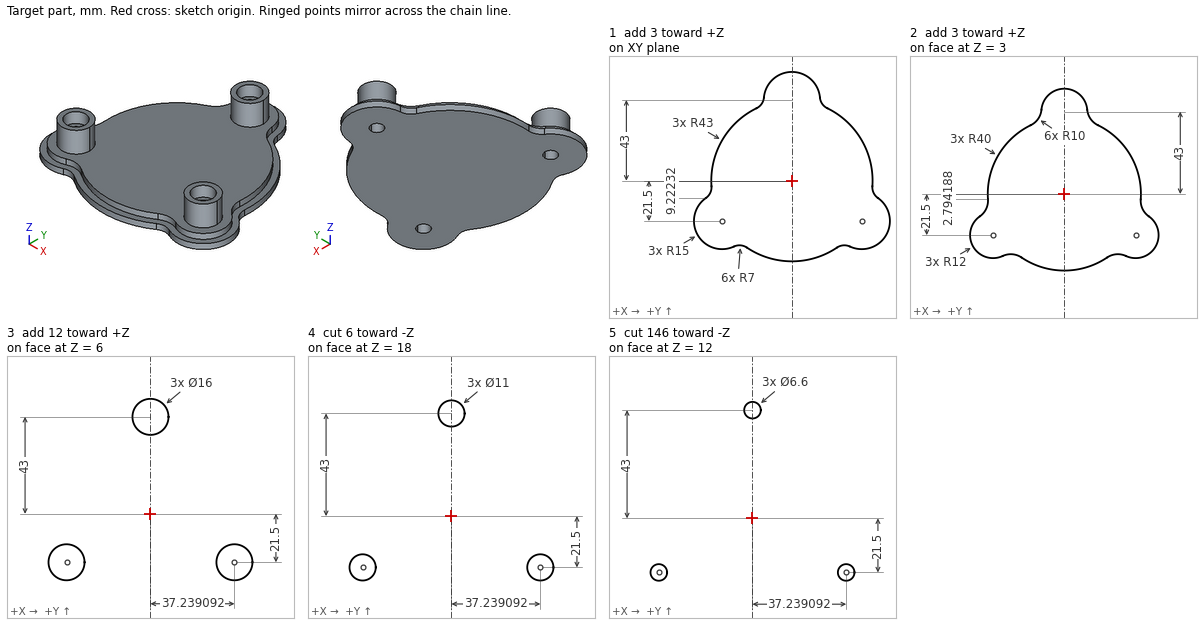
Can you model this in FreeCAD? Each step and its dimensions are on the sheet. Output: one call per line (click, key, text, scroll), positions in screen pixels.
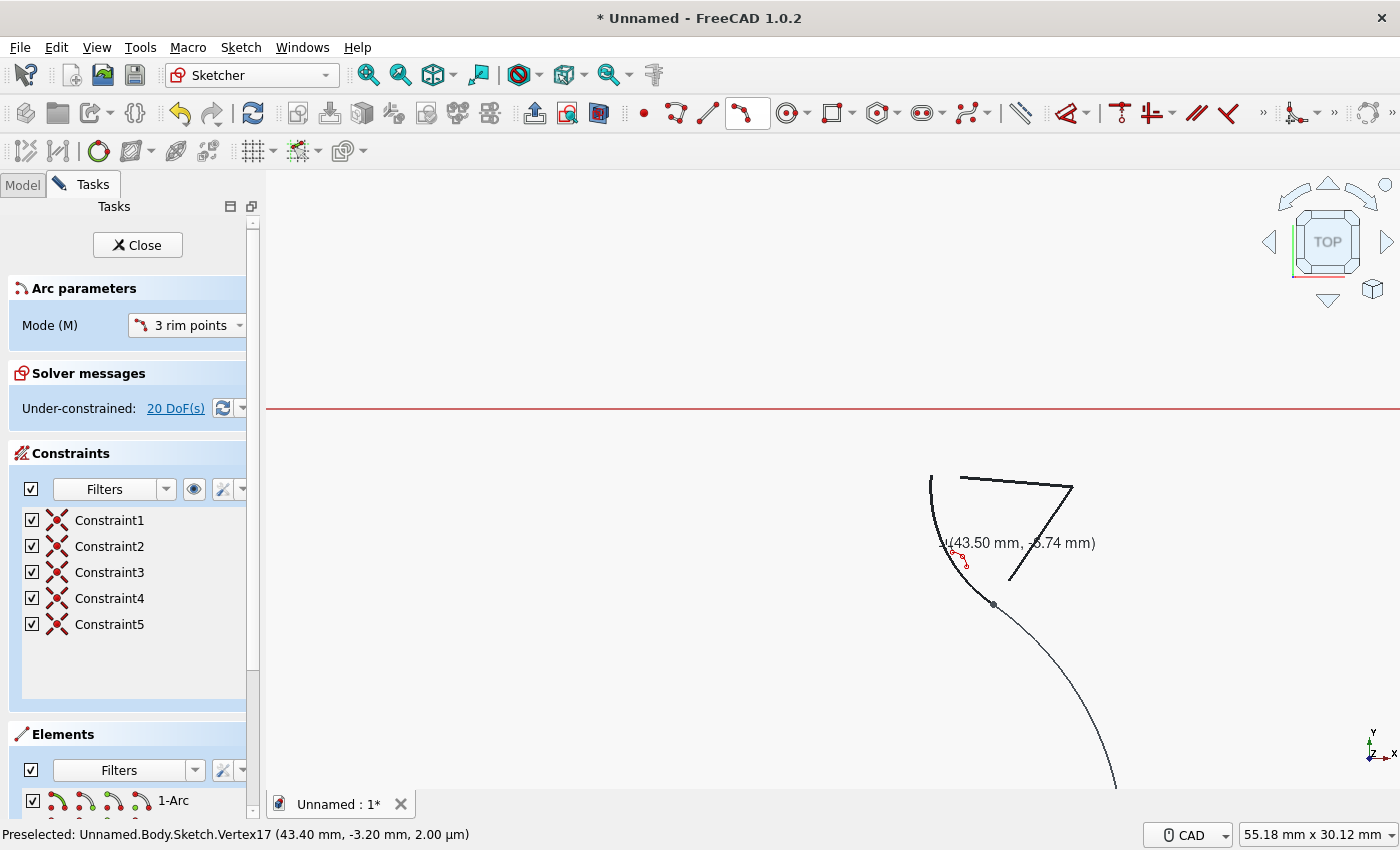
click(946, 543)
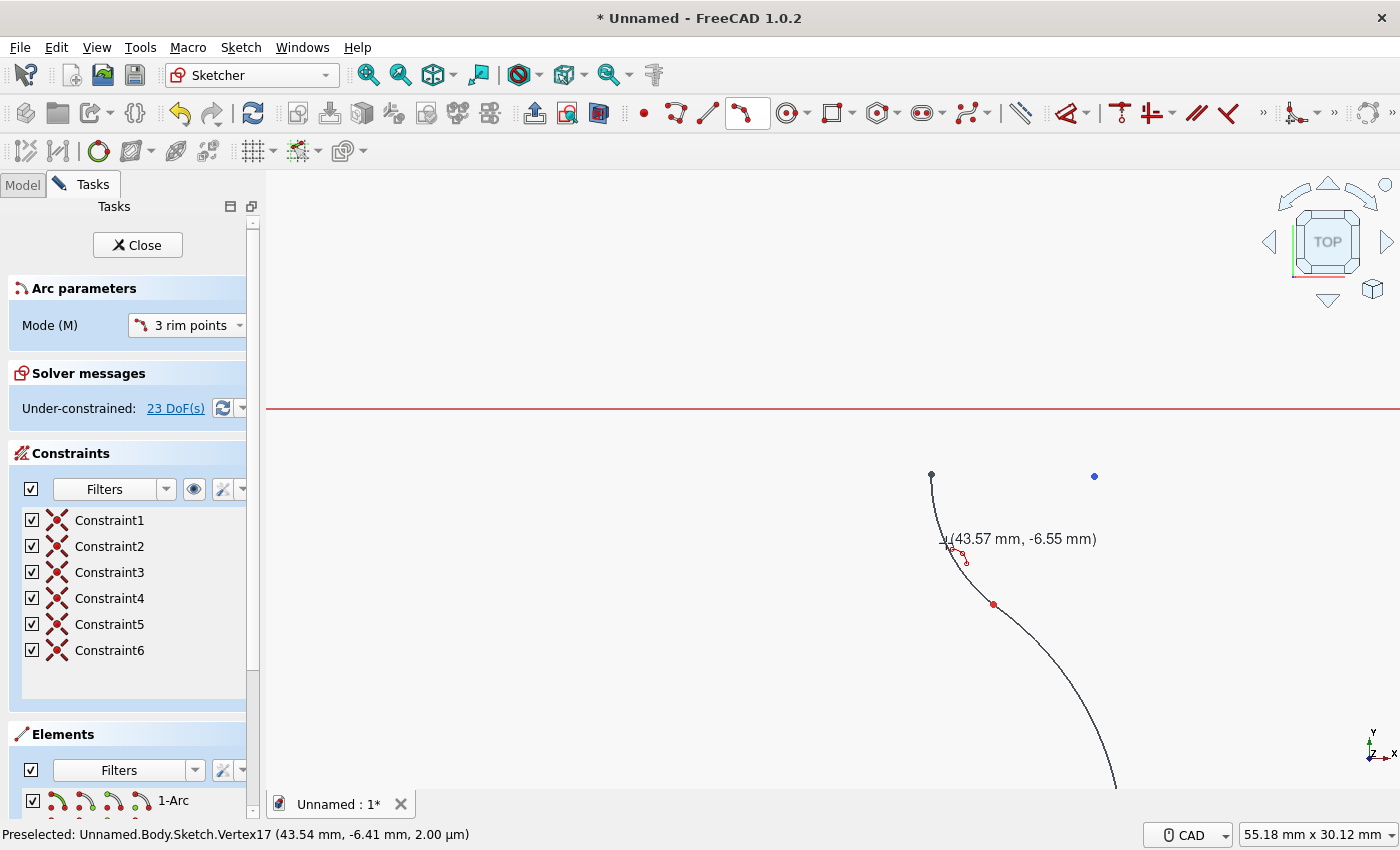
scroll(945, 536, down, 8)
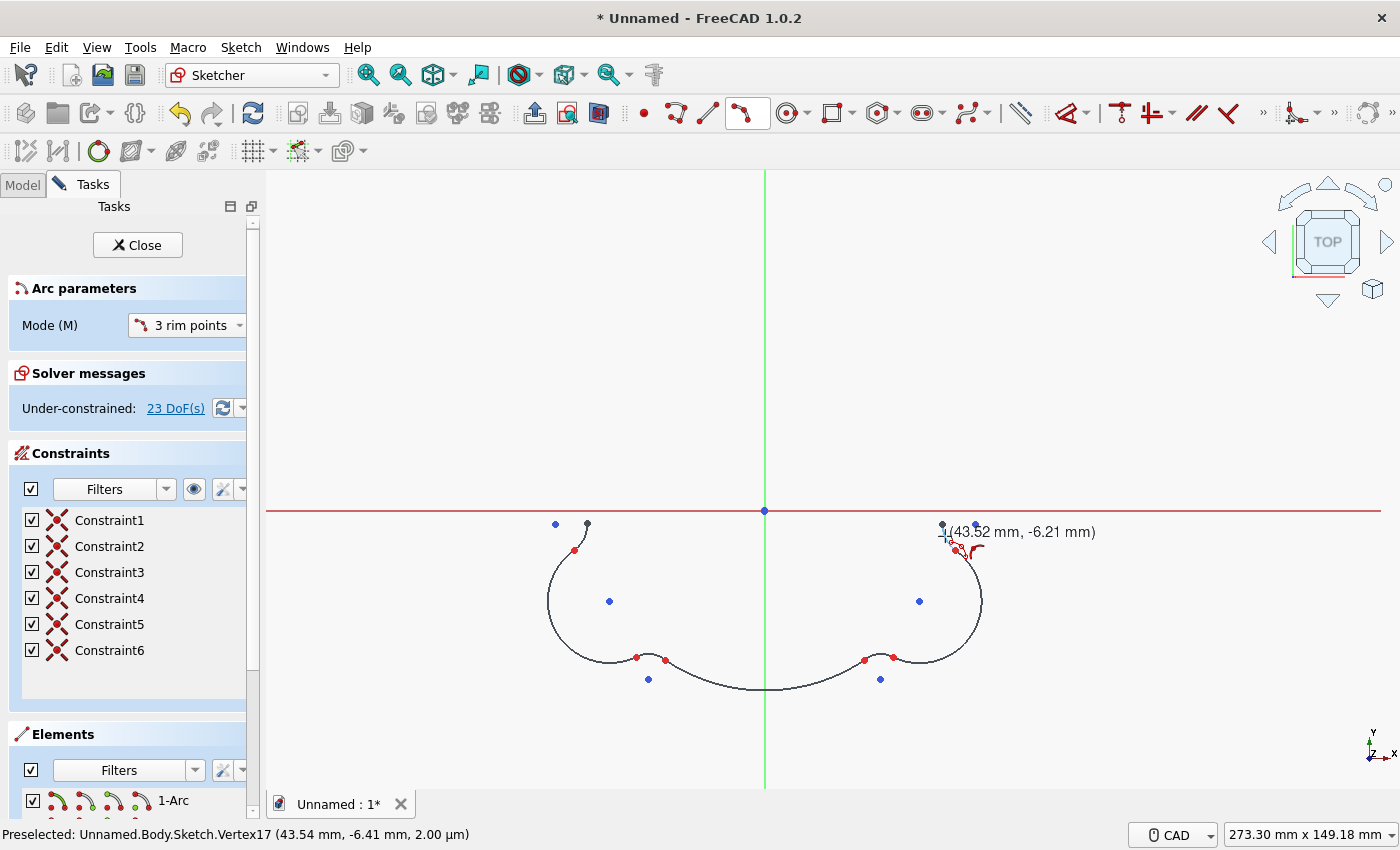
scroll(943, 523, up, 2)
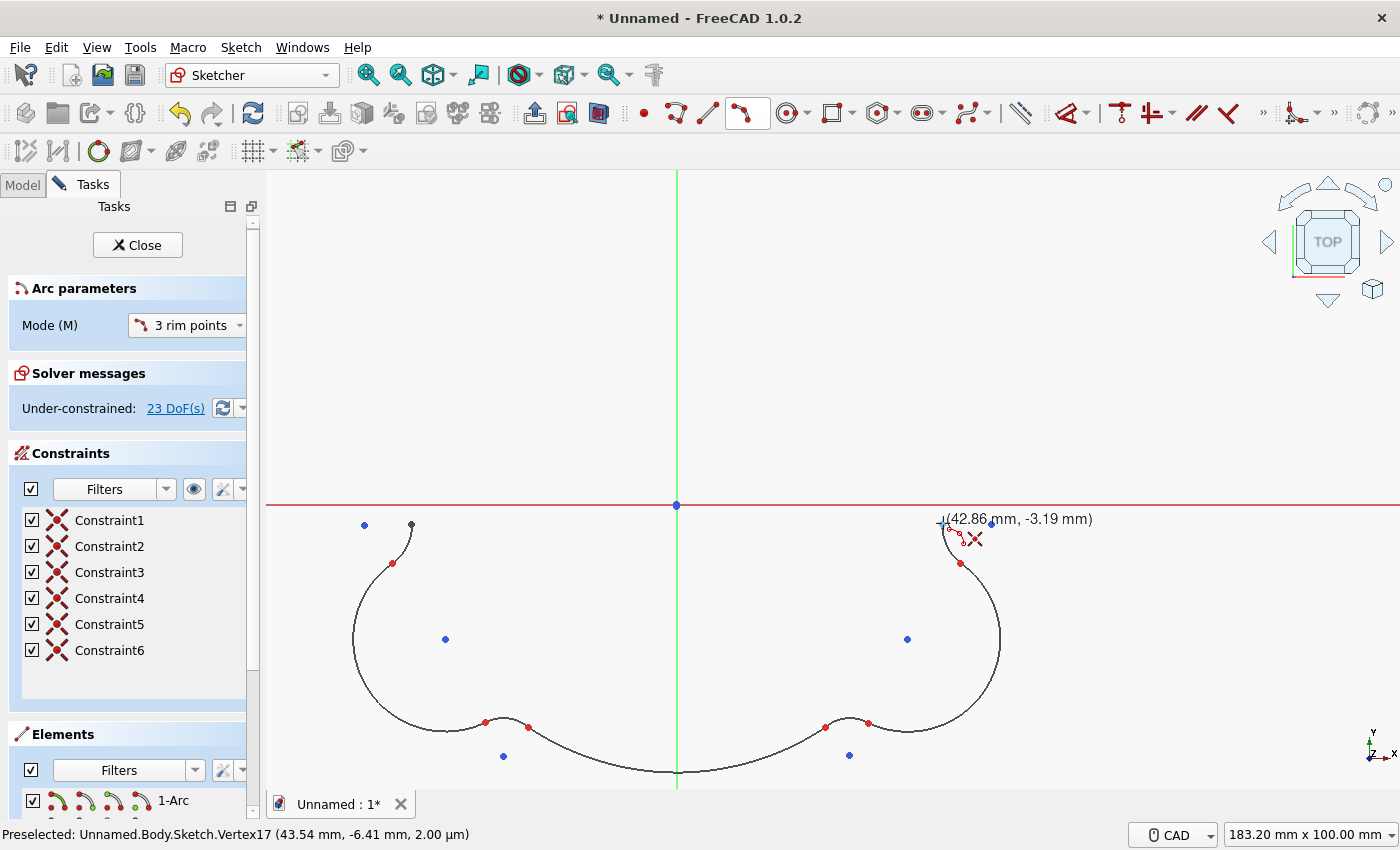
click(942, 524)
click(794, 265)
click(908, 372)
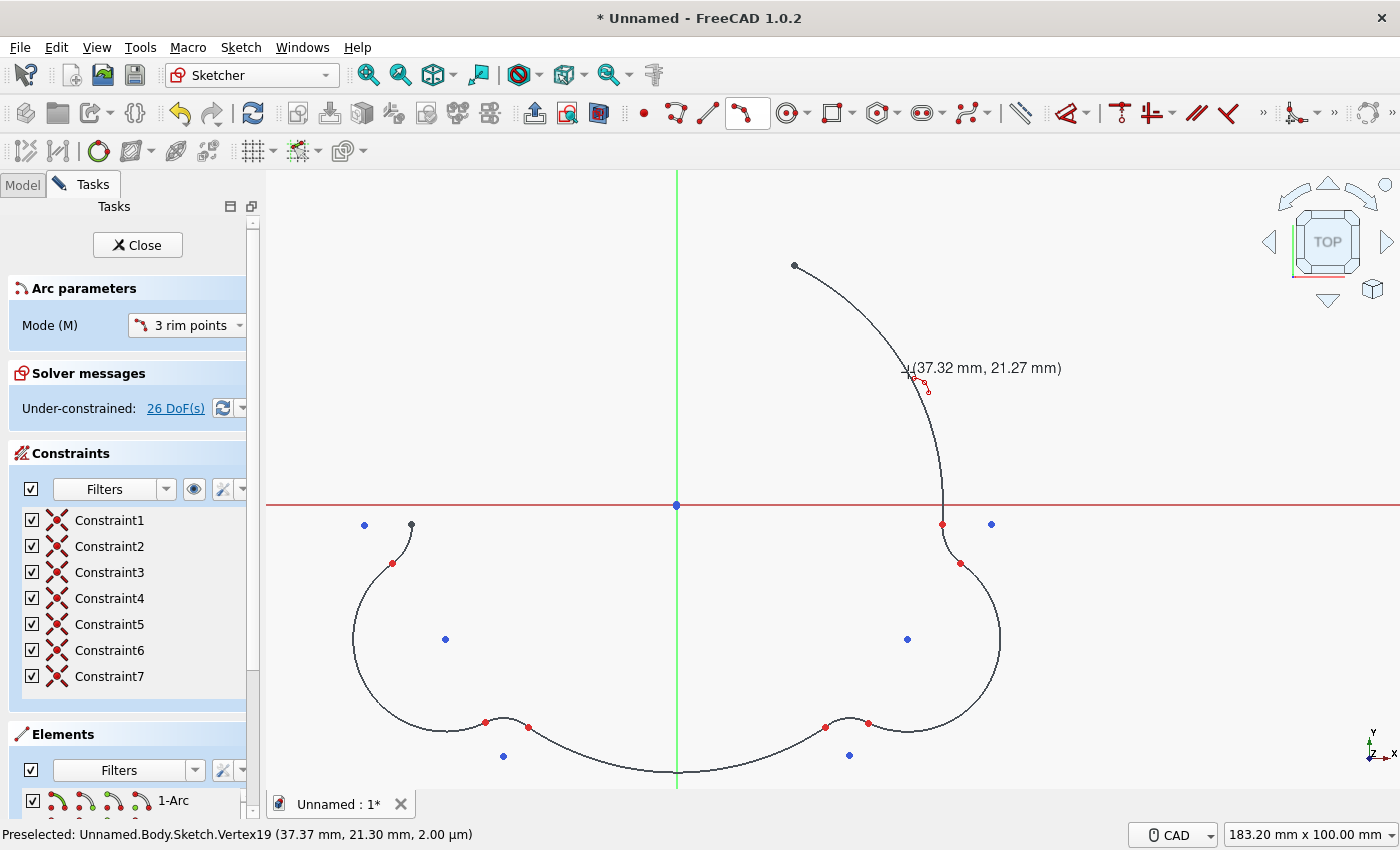
click(794, 266)
click(769, 230)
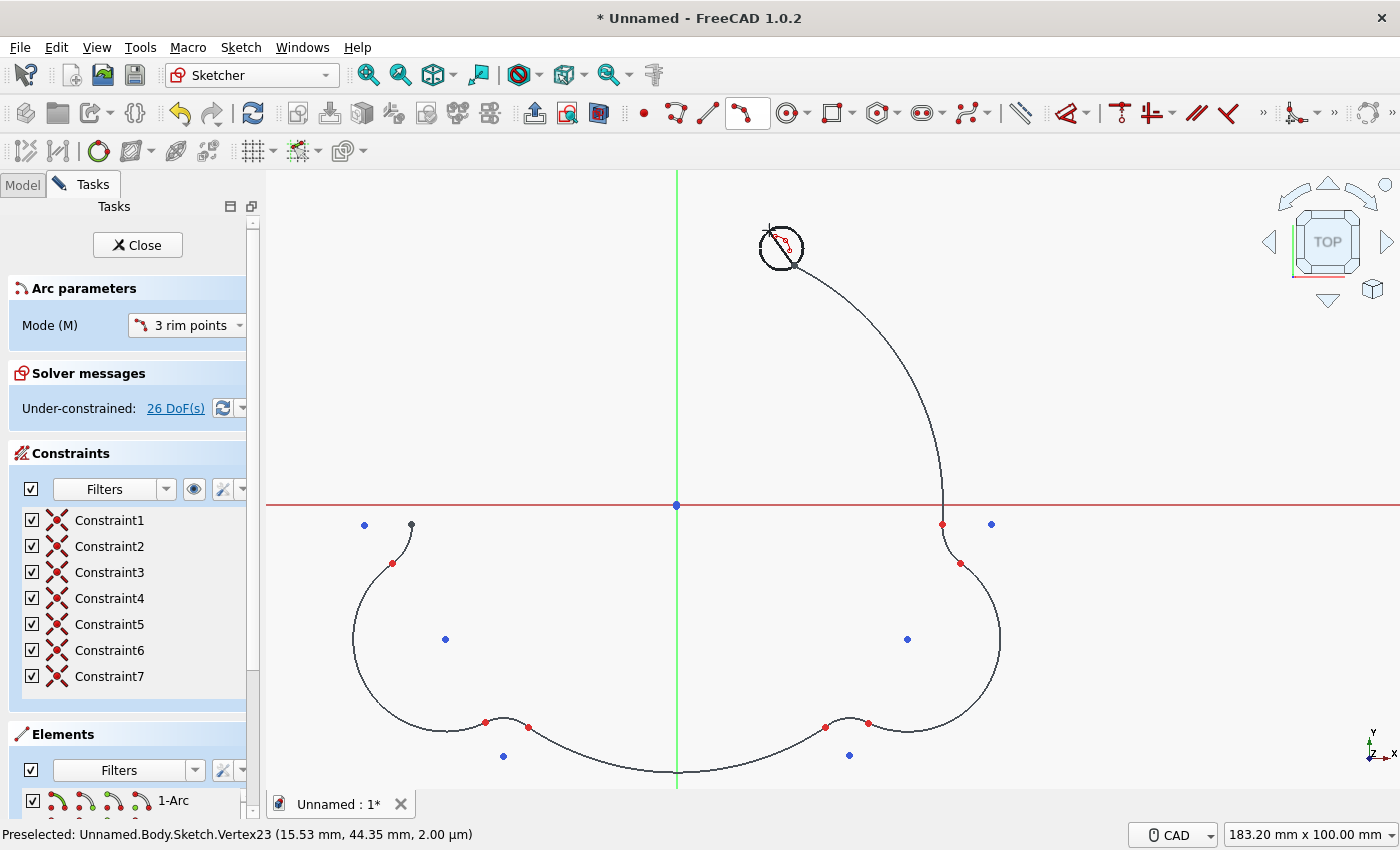
scroll(777, 251, up, 6)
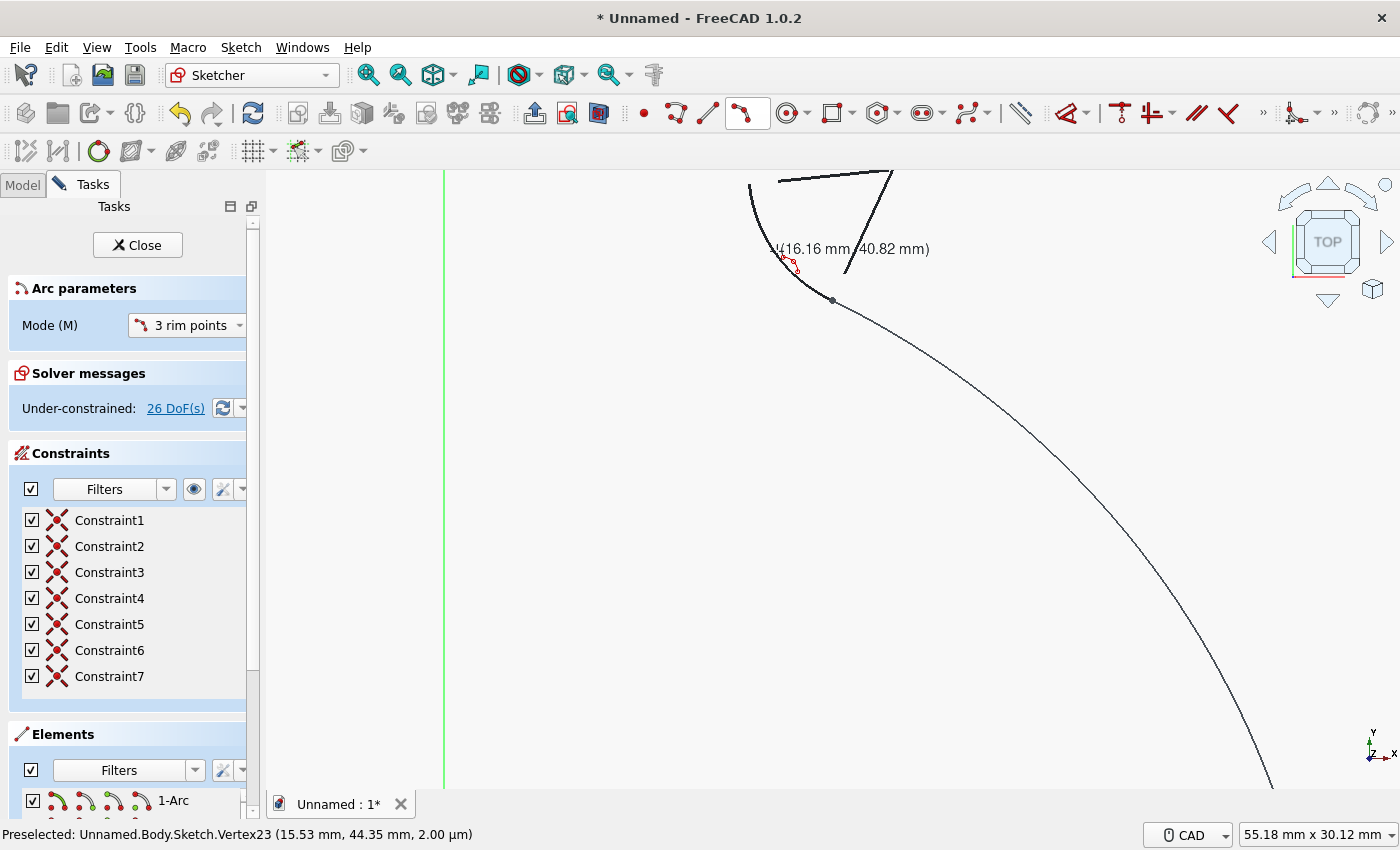
click(776, 251)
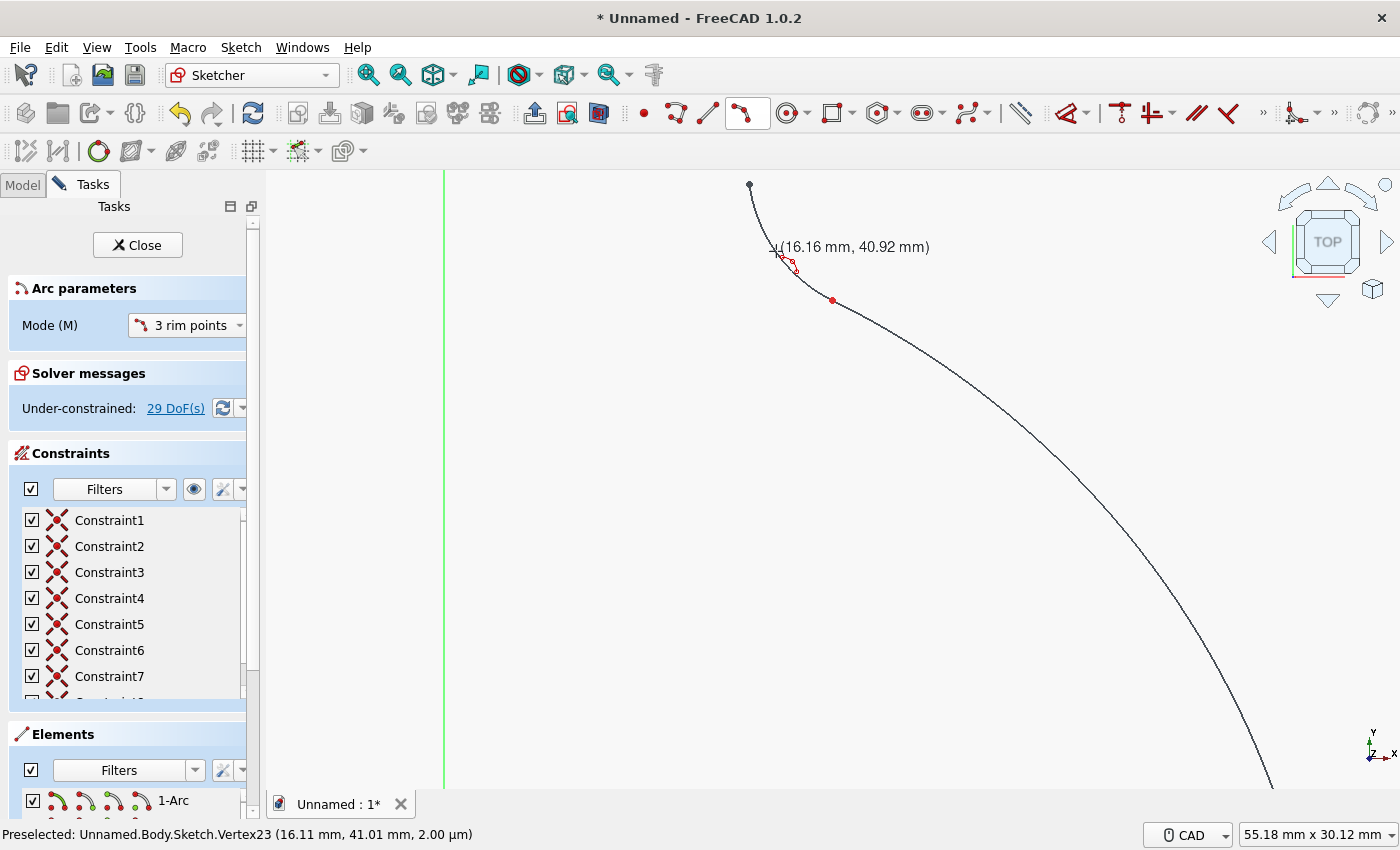
scroll(846, 363, down, 8)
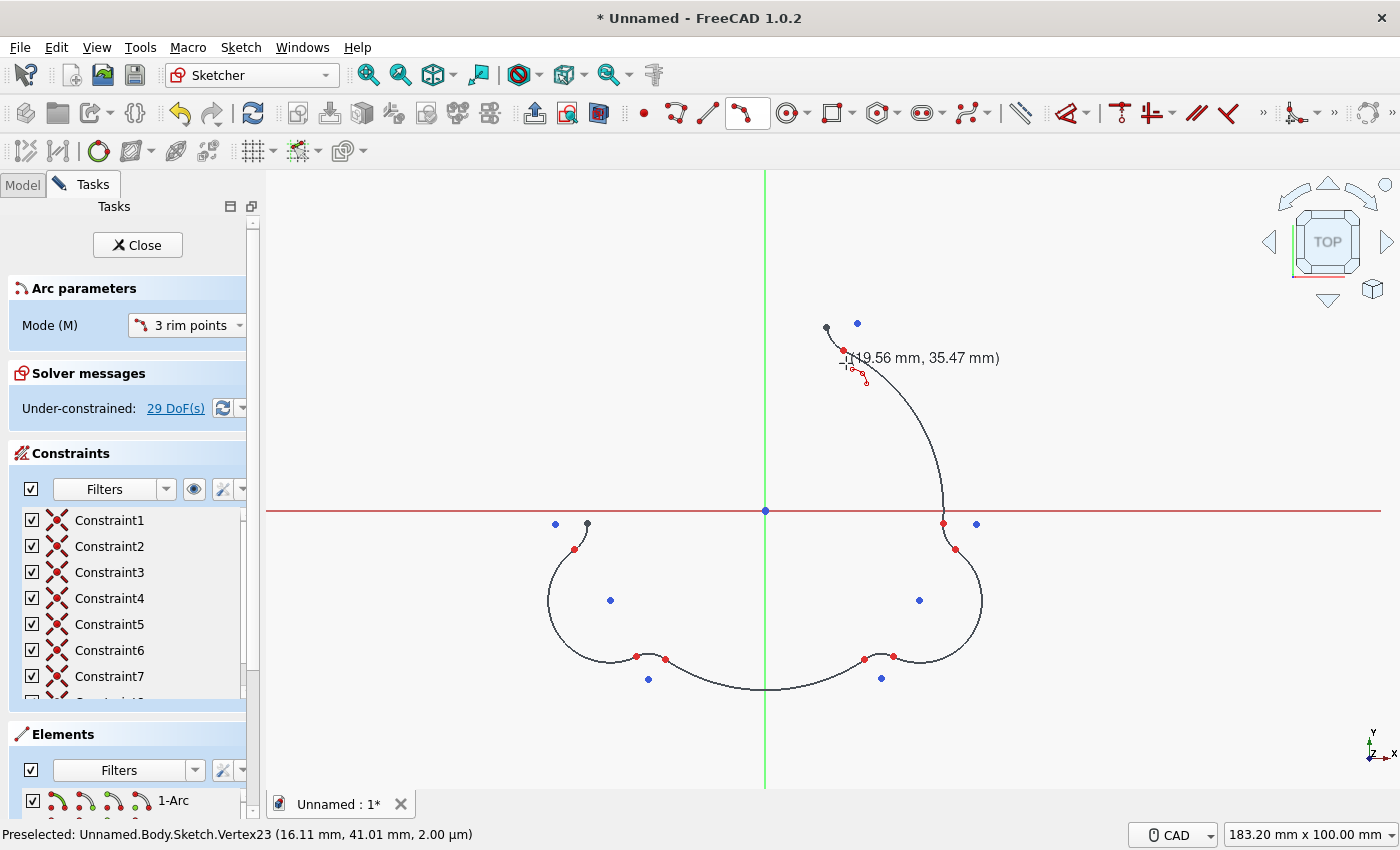
click(827, 327)
click(703, 327)
click(783, 273)